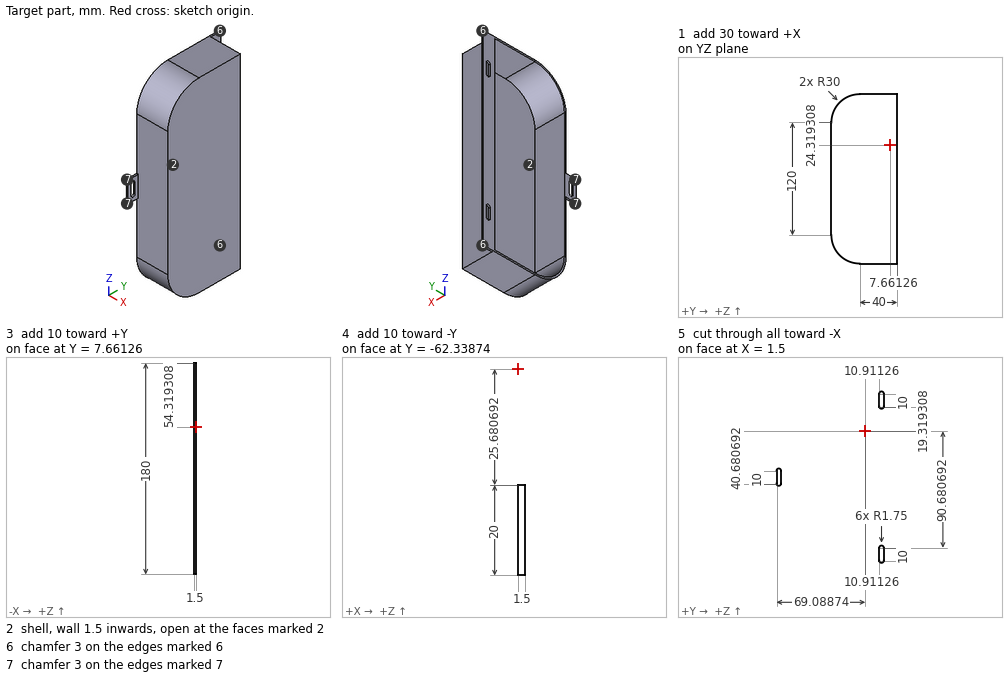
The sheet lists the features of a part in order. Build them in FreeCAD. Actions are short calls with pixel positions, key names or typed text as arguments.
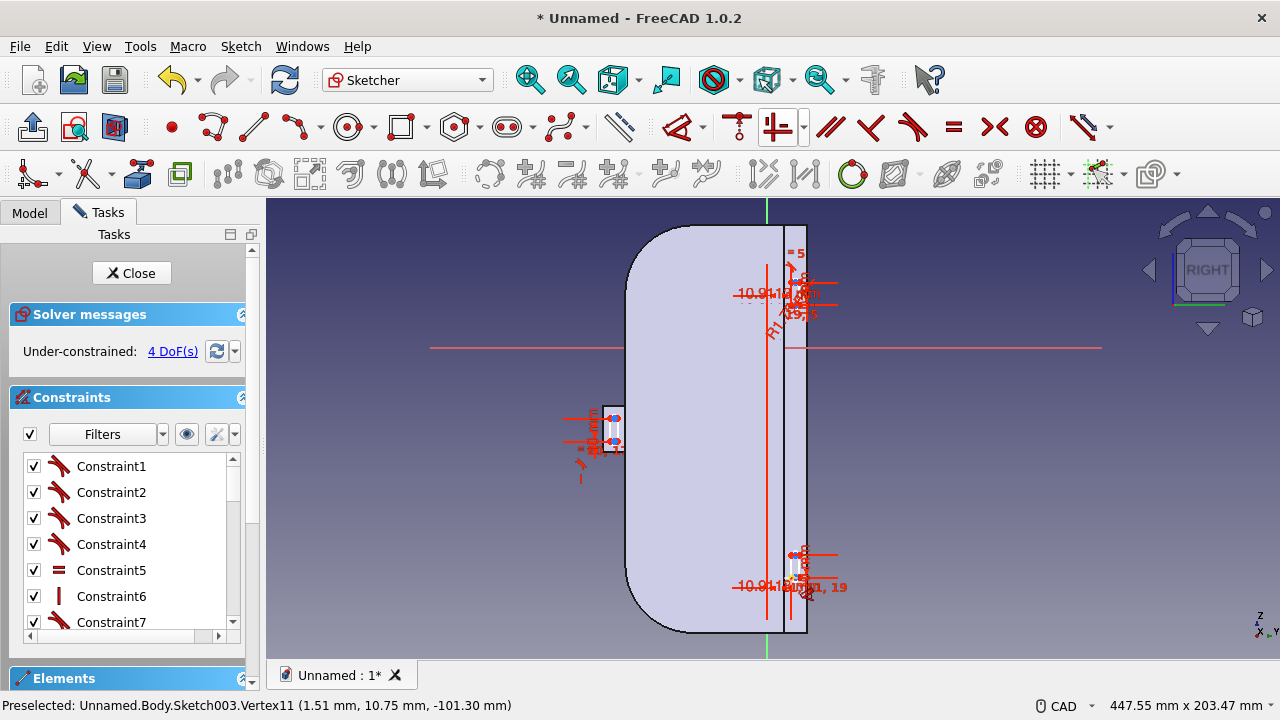
scroll(610, 442, up, 6)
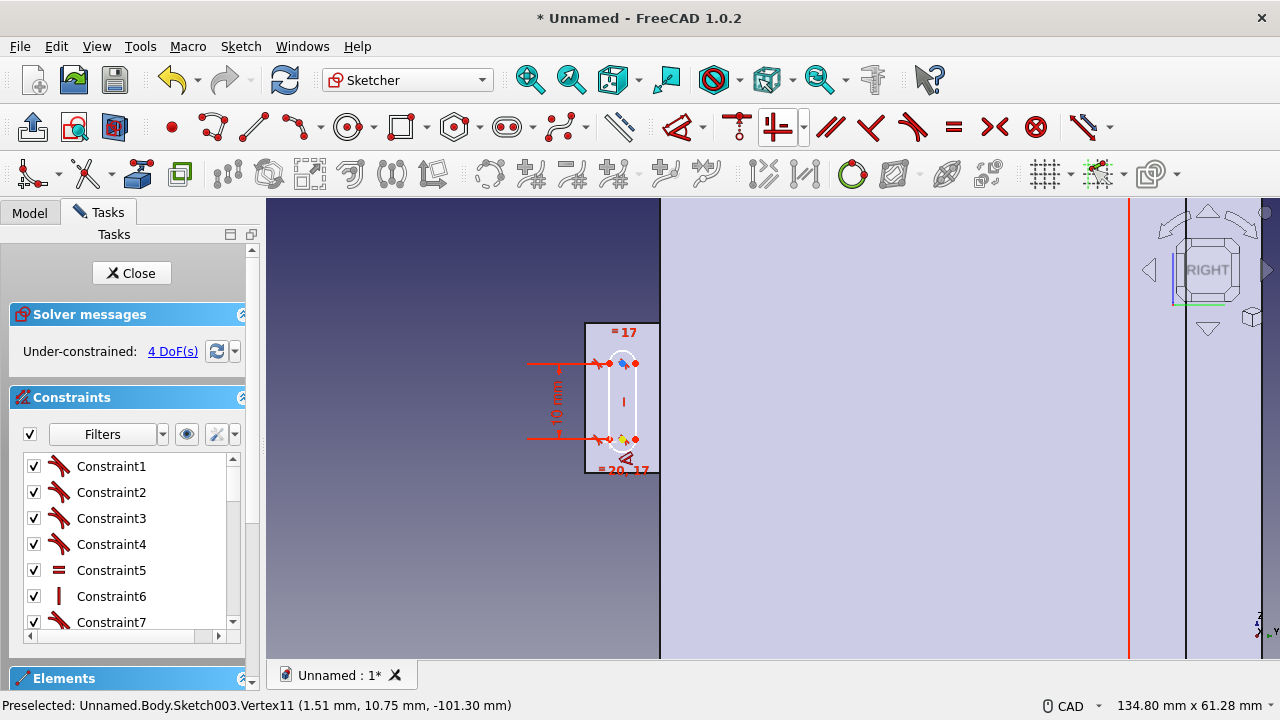
click(609, 439)
click(862, 473)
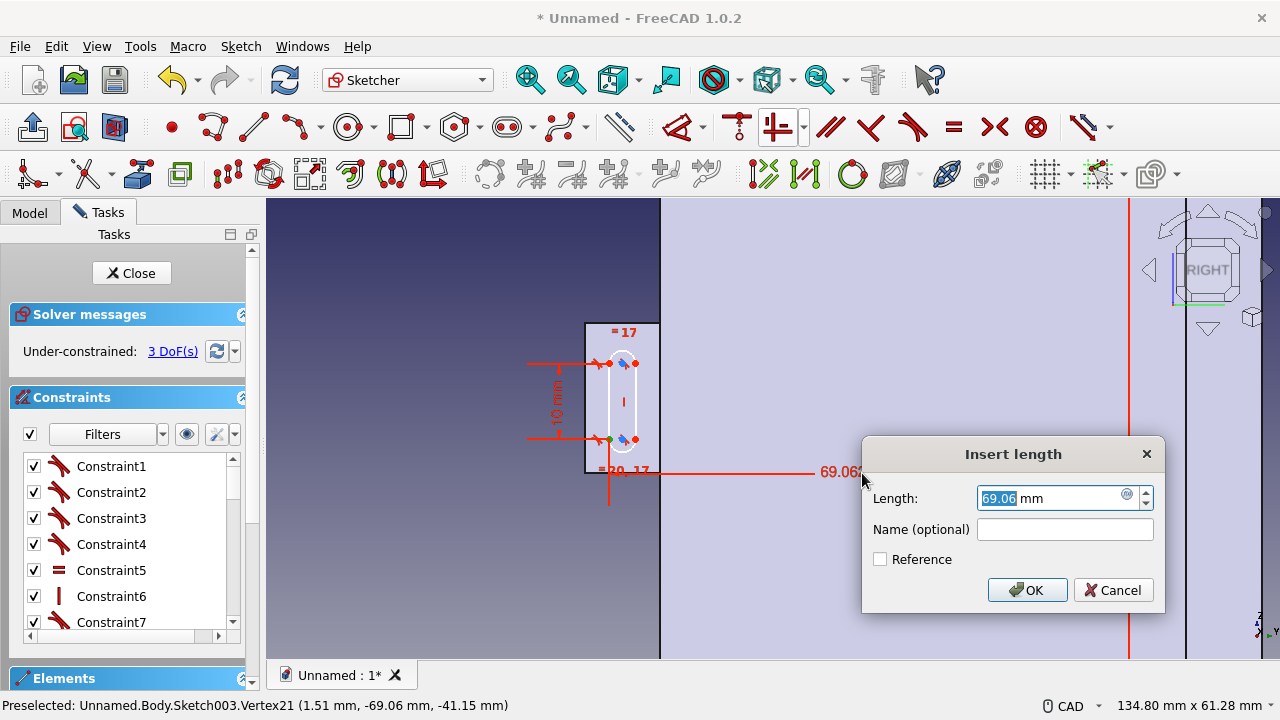
text(69.08874)
key(Return)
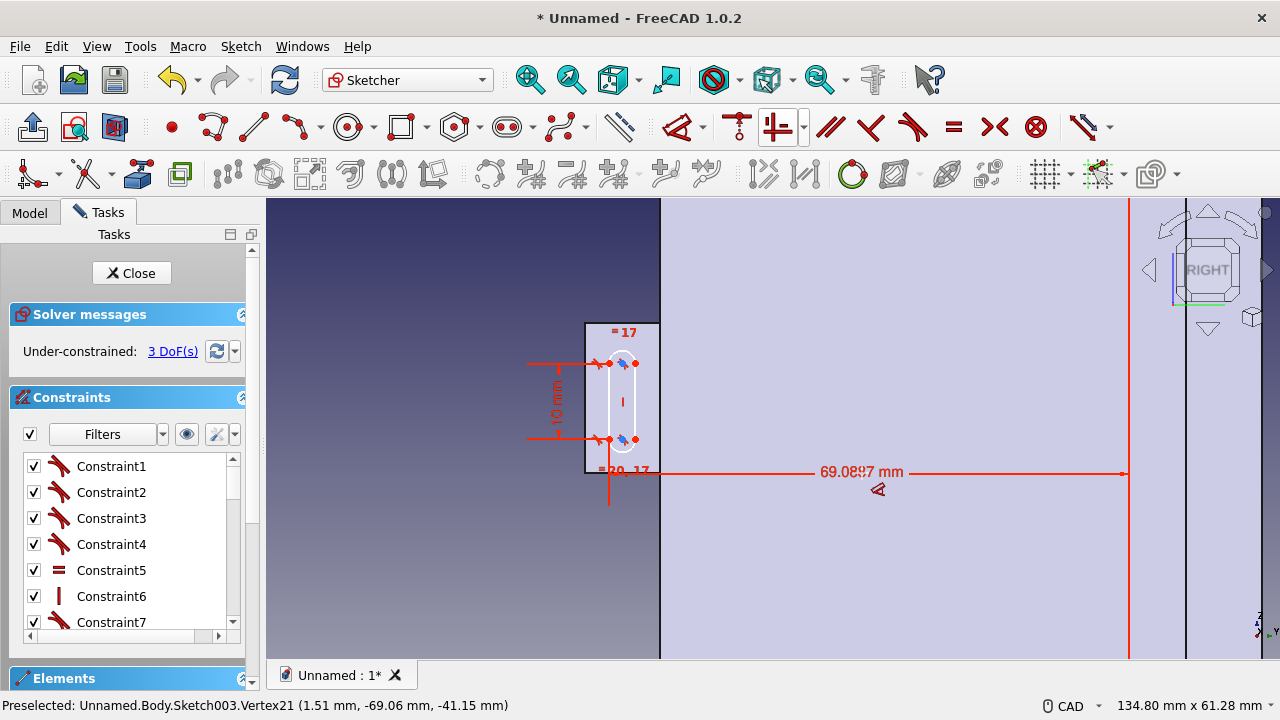
scroll(610, 442, down, 6)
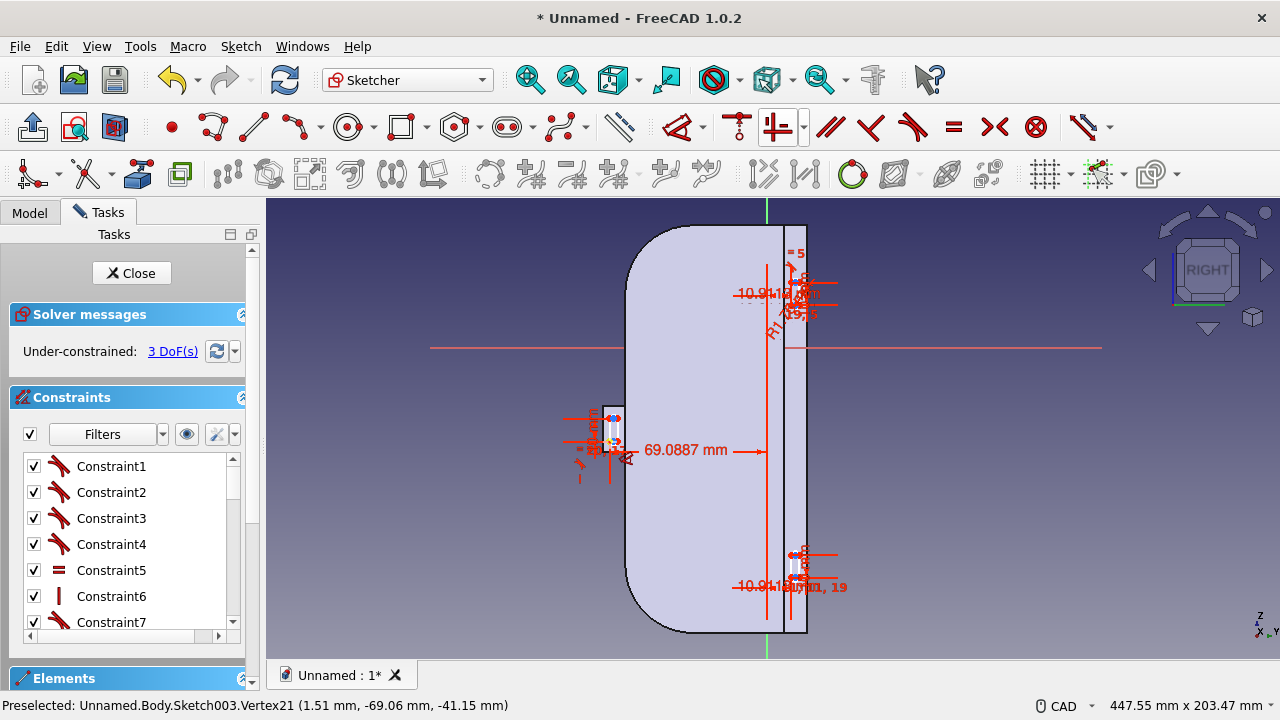
scroll(791, 305, up, 6)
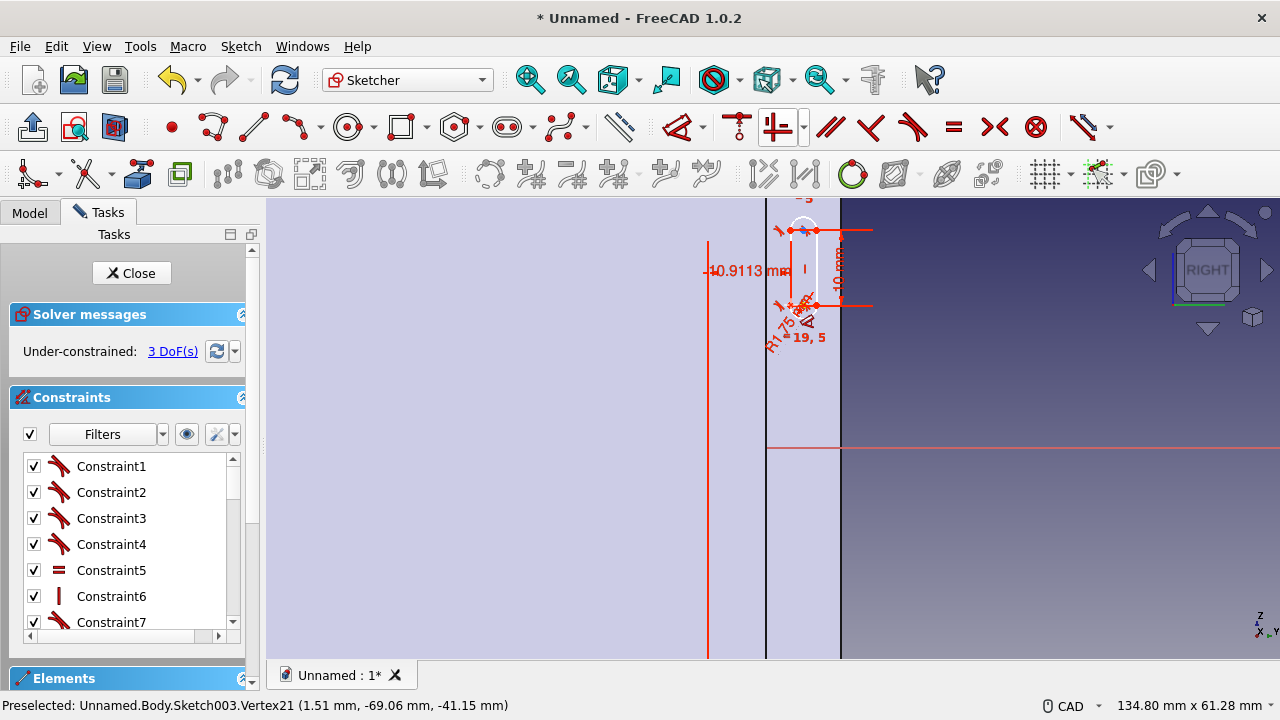
click(791, 306)
click(825, 377)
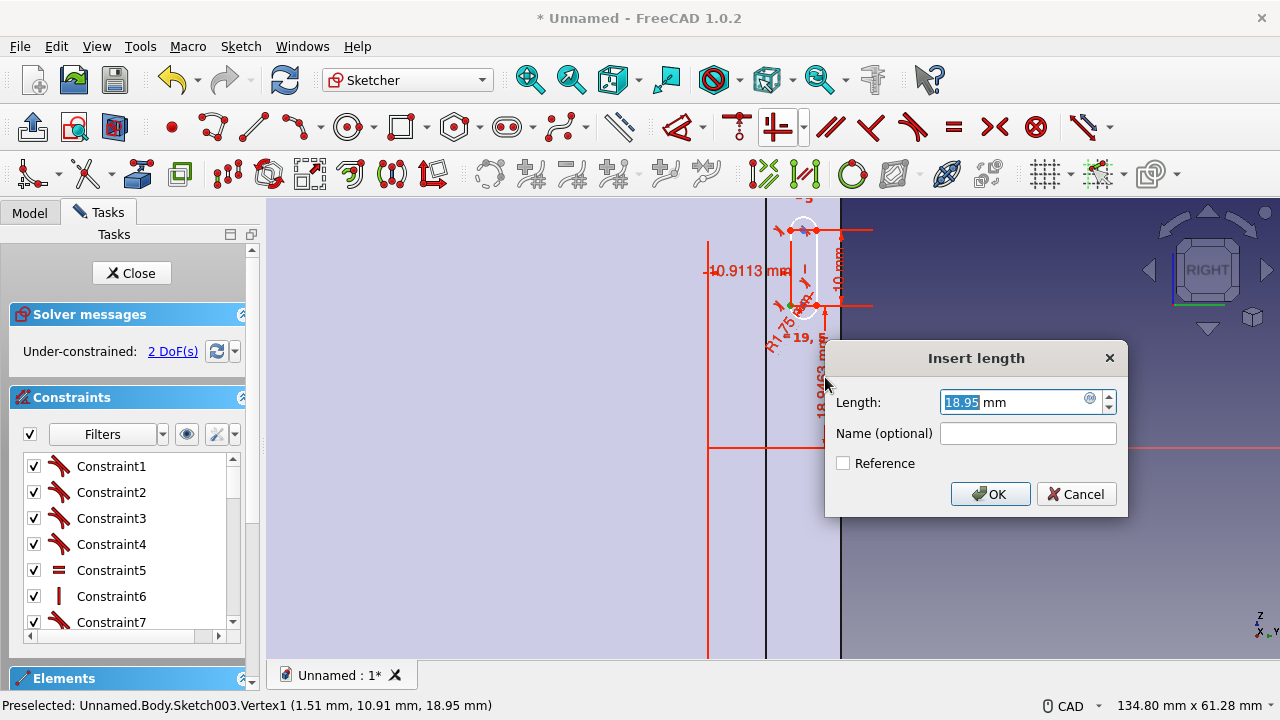
text(19.319308)
key(Return)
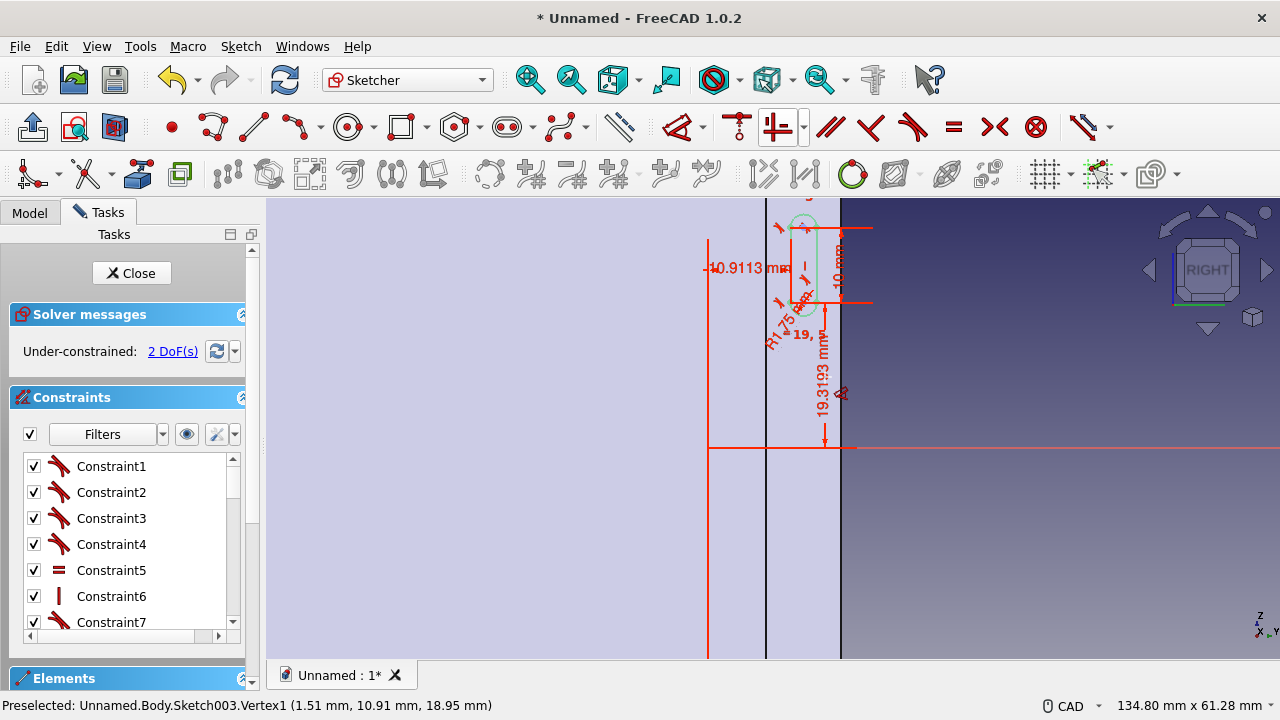
scroll(791, 304, down, 6)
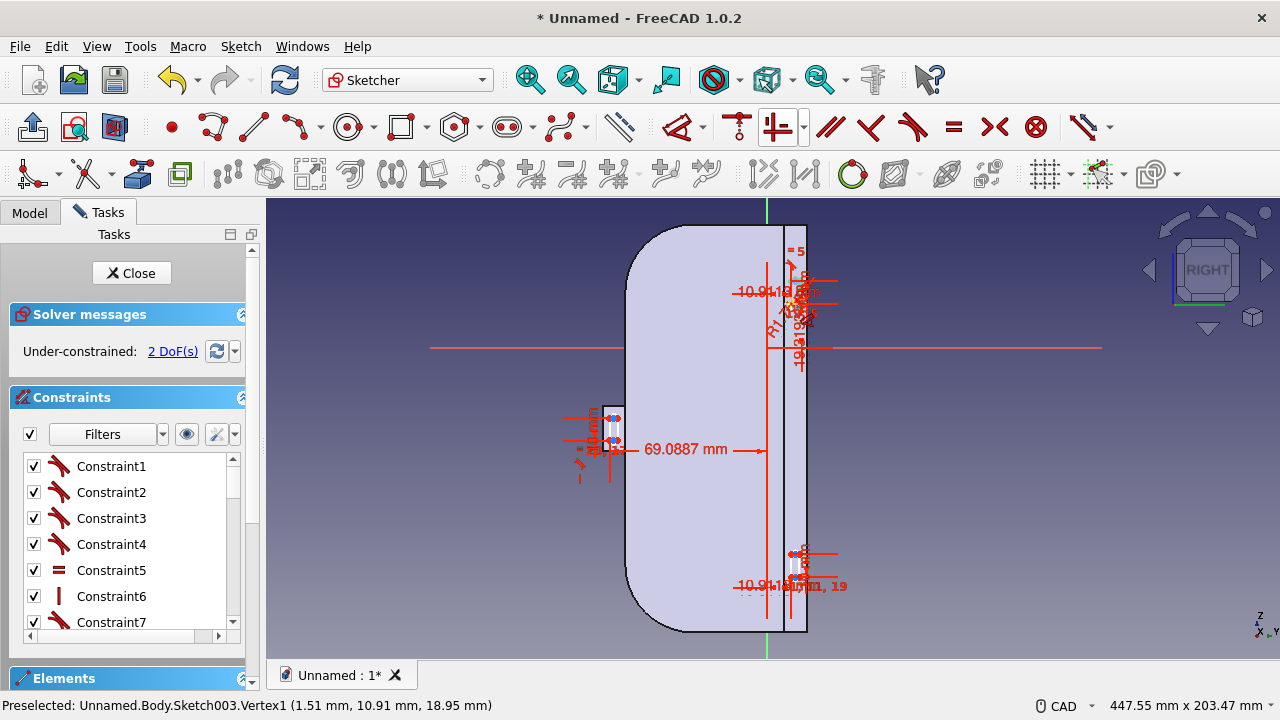
scroll(799, 554, up, 6)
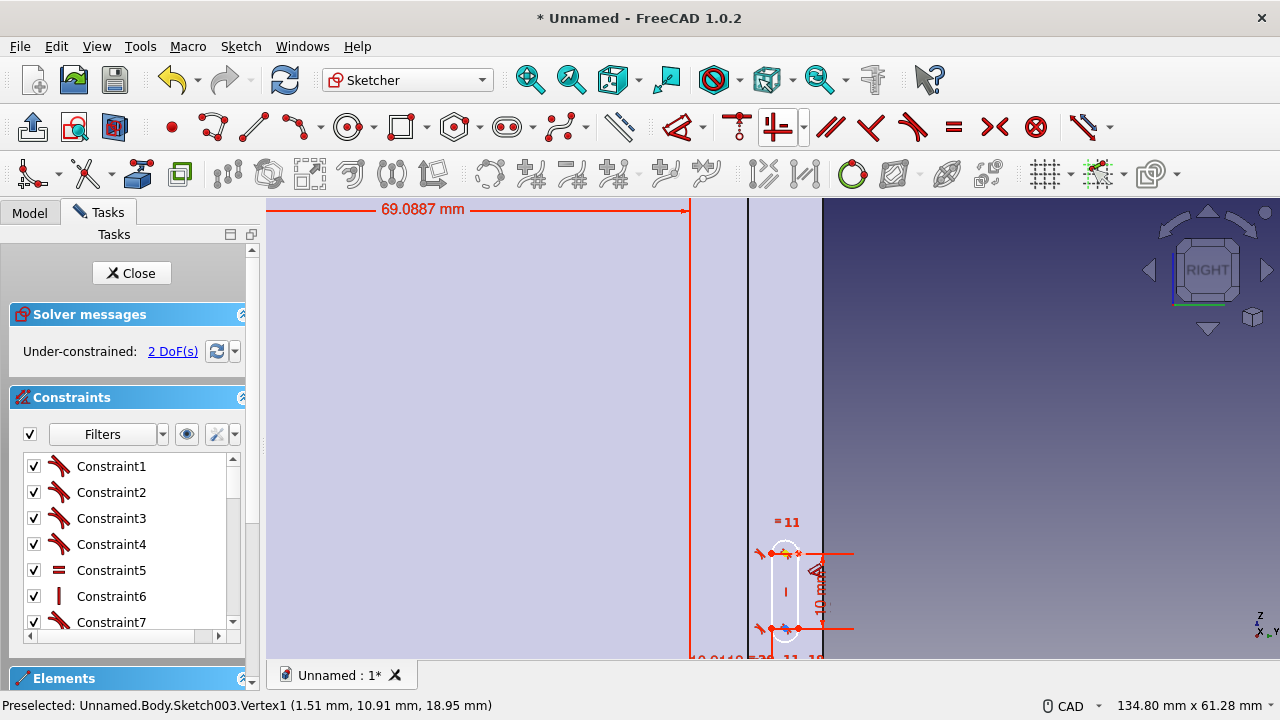
click(798, 554)
click(832, 390)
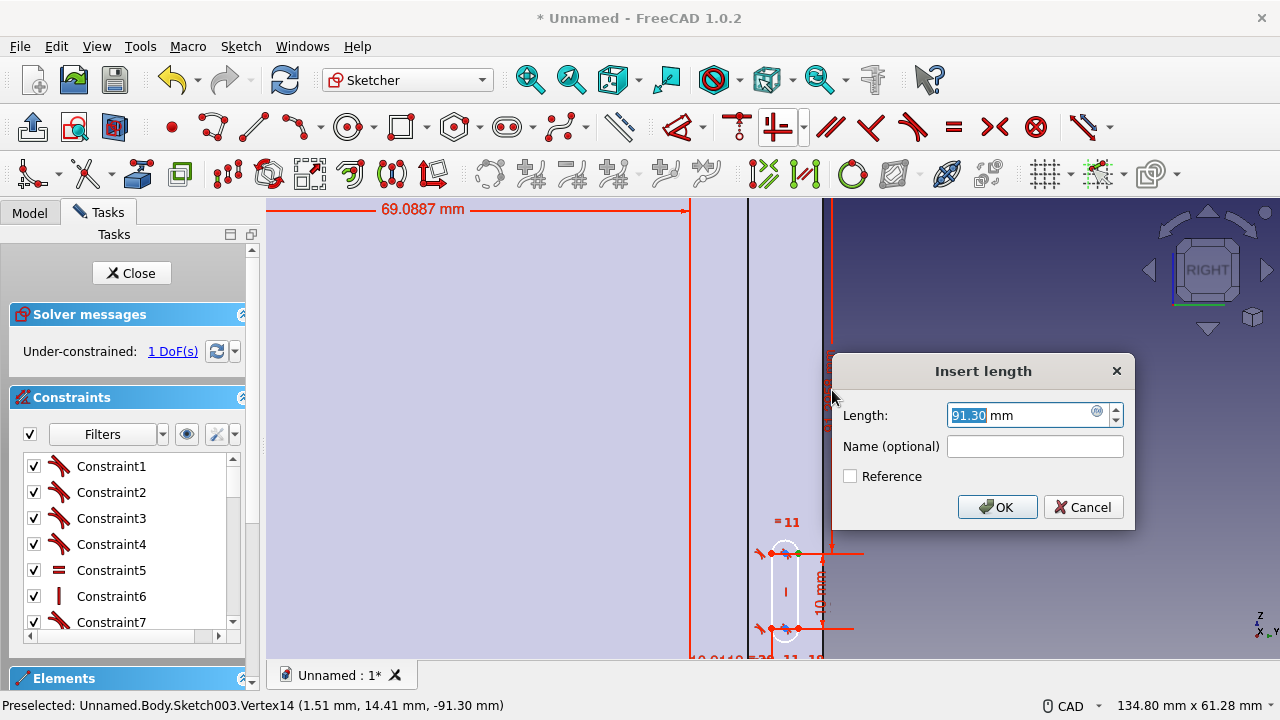
text(90.680692)
key(Return)